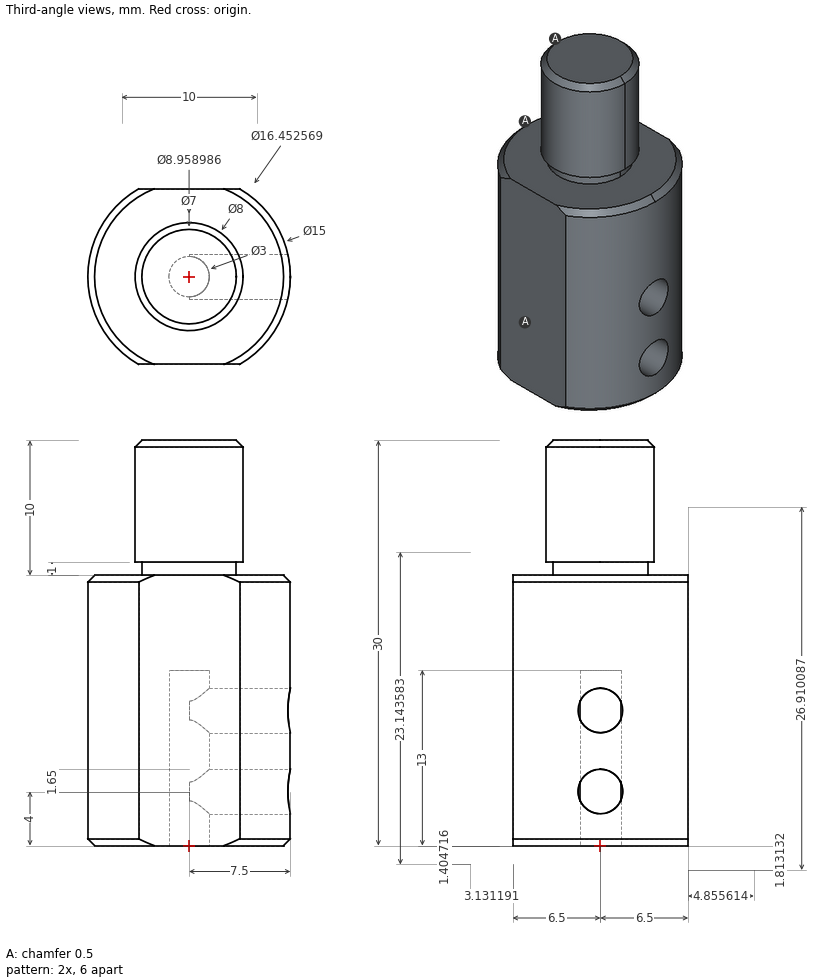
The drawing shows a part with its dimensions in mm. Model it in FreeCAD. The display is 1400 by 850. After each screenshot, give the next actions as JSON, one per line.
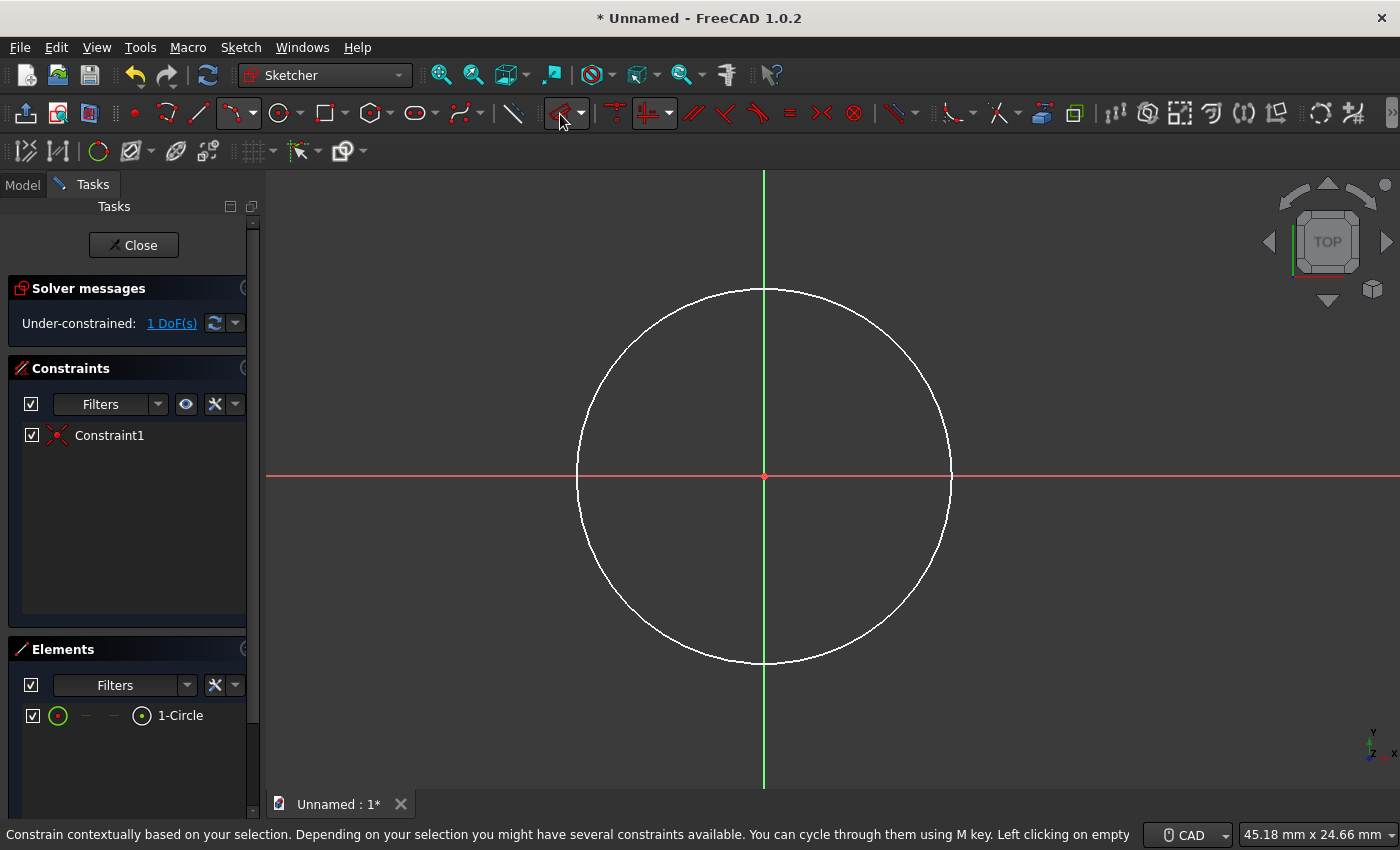
{"action": "left_click", "coordinate": [896, 343]}
{"action": "left_click", "coordinate": [918, 320]}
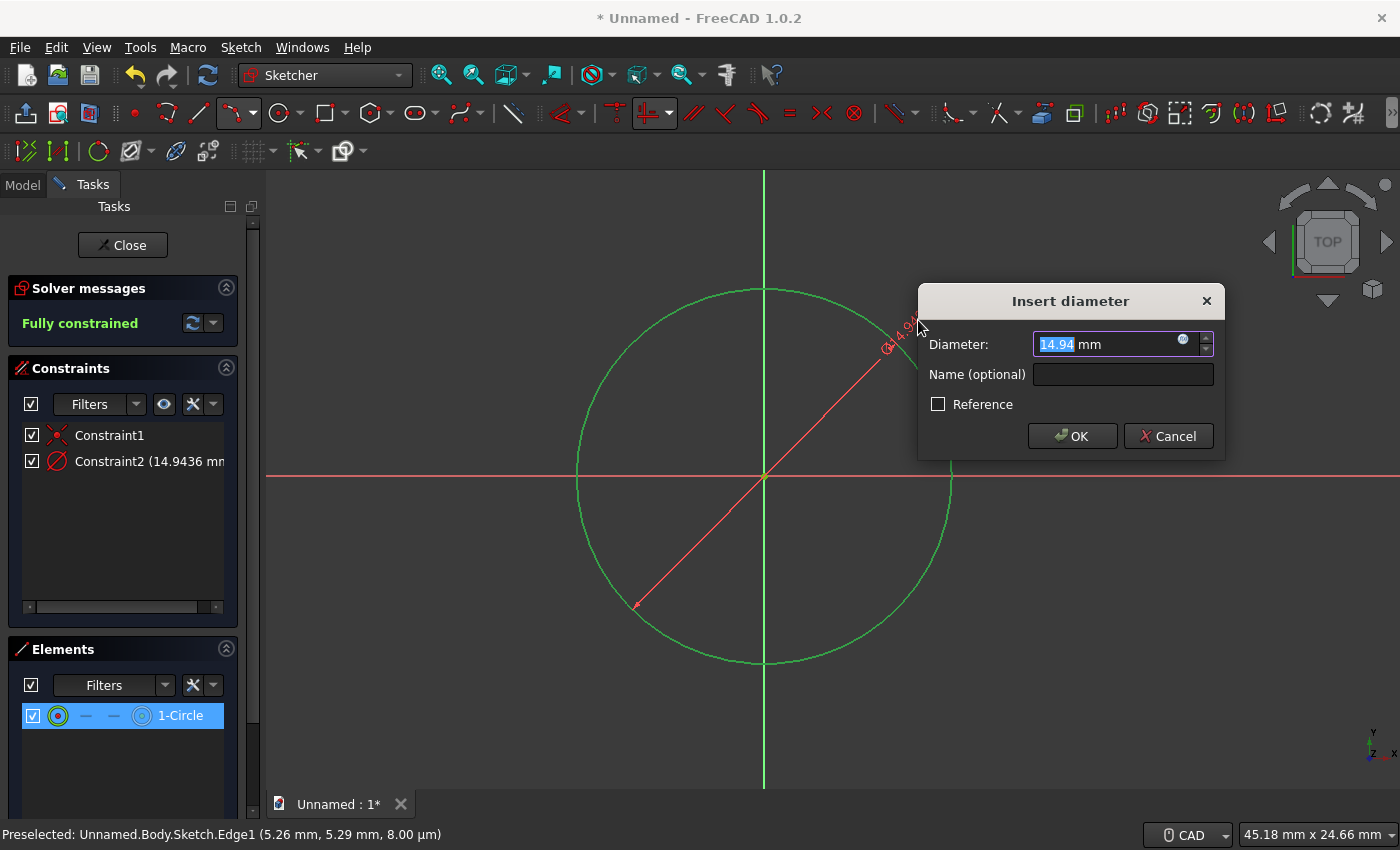
{"action": "type", "text": "15"}
{"action": "key", "text": "Return"}
{"action": "key", "text": "Escape"}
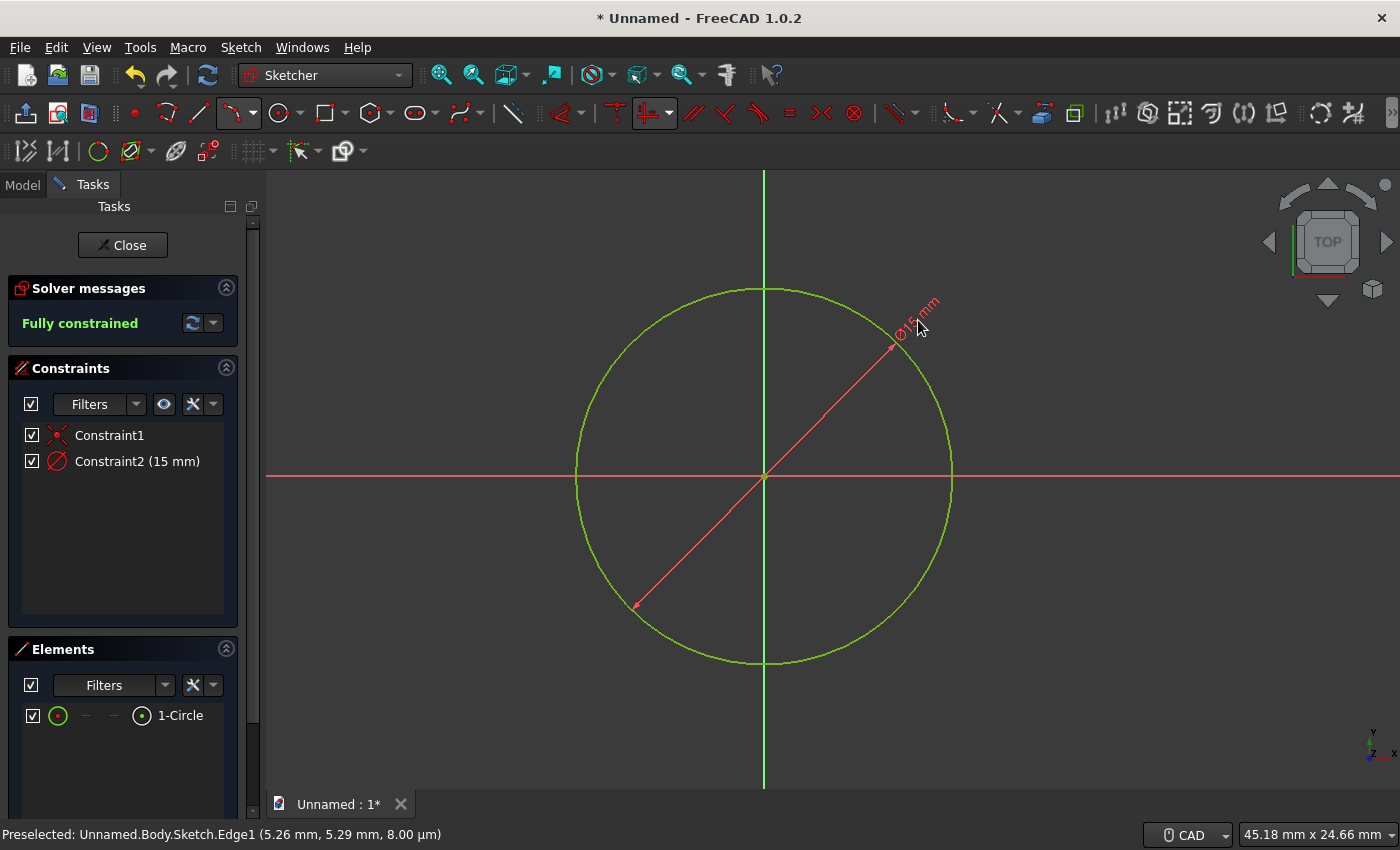
{"action": "left_click", "coordinate": [123, 245]}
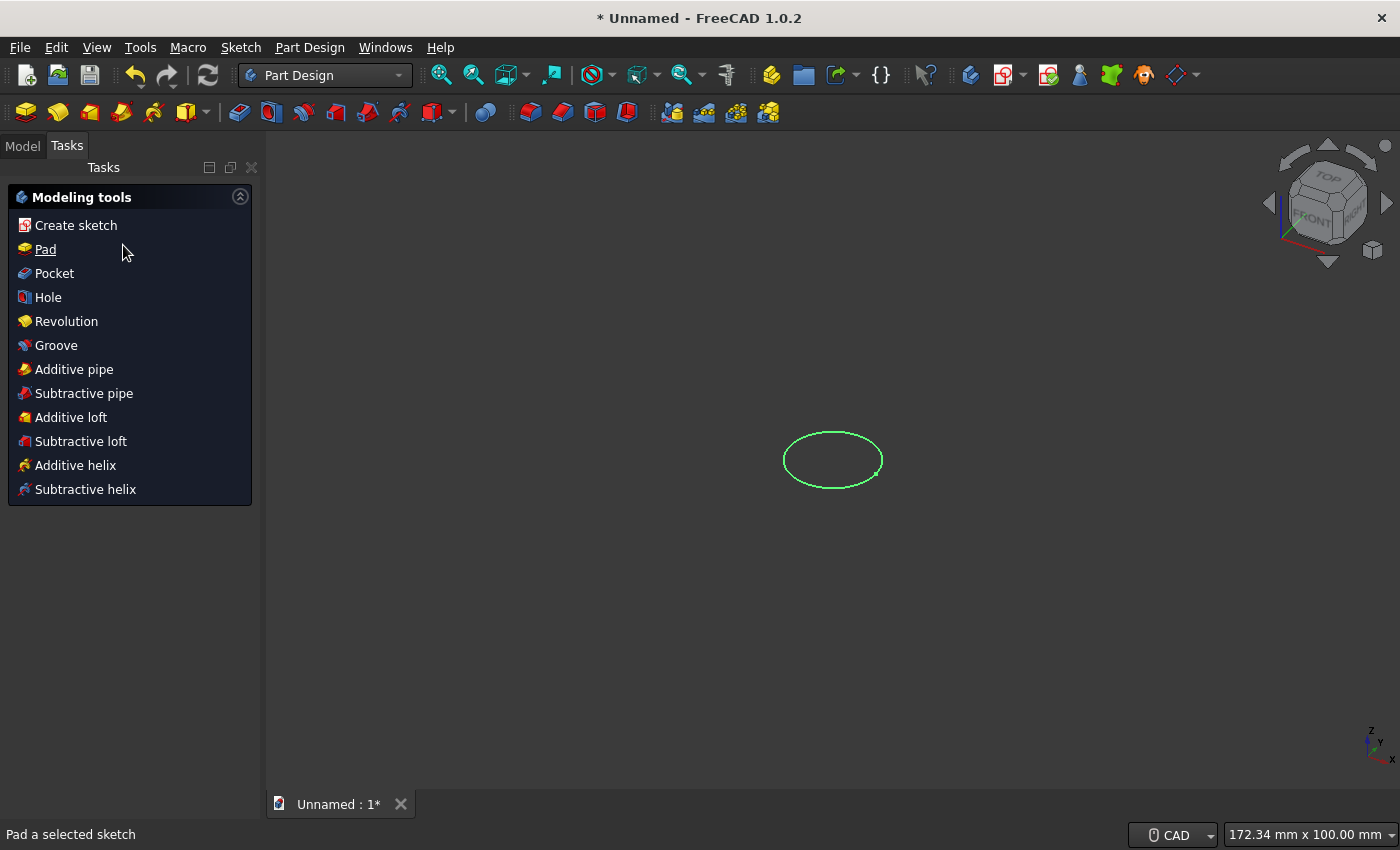
{"action": "left_click", "coordinate": [26, 112]}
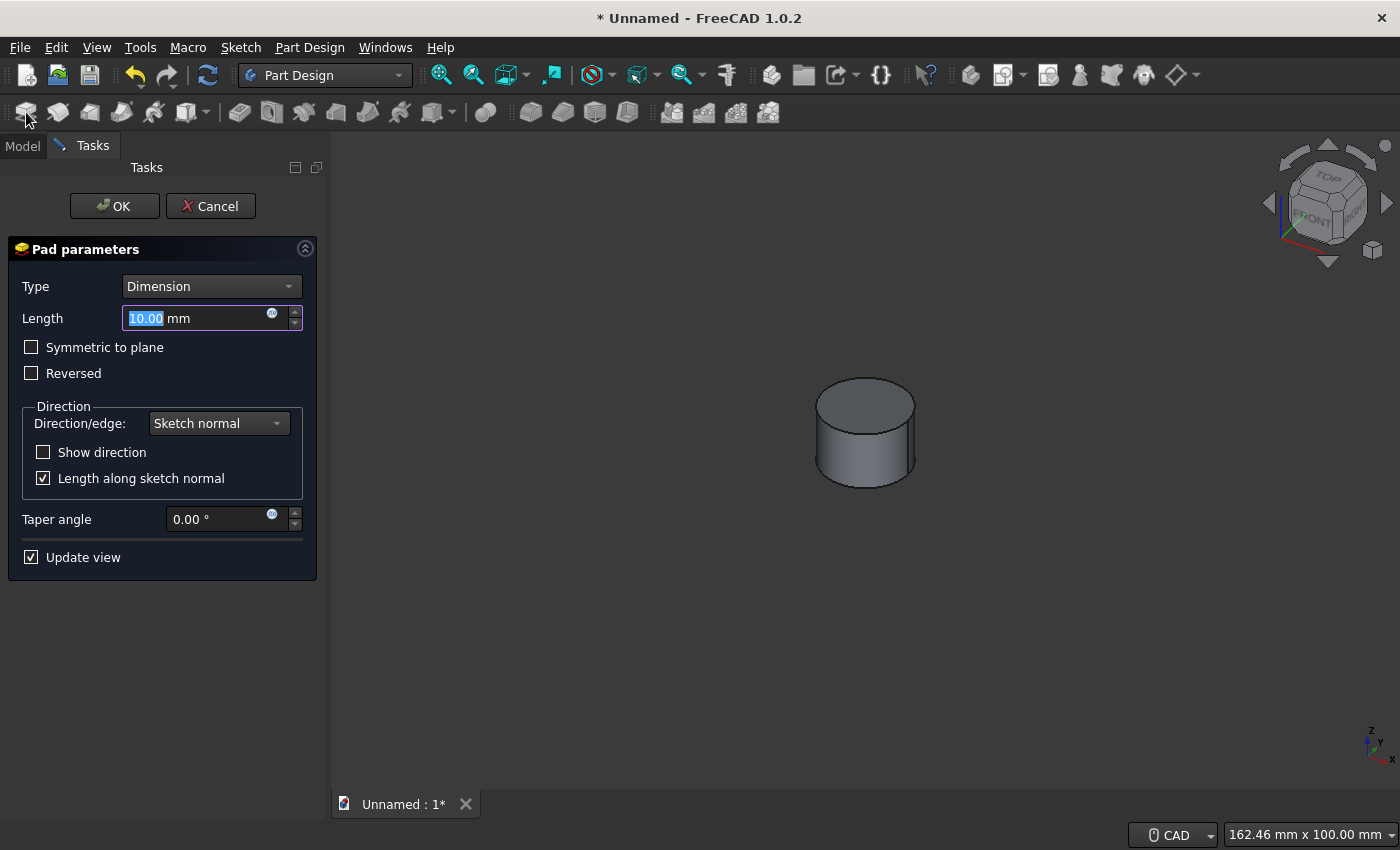
{"action": "type", "text": "30"}
{"action": "key", "text": "Tab"}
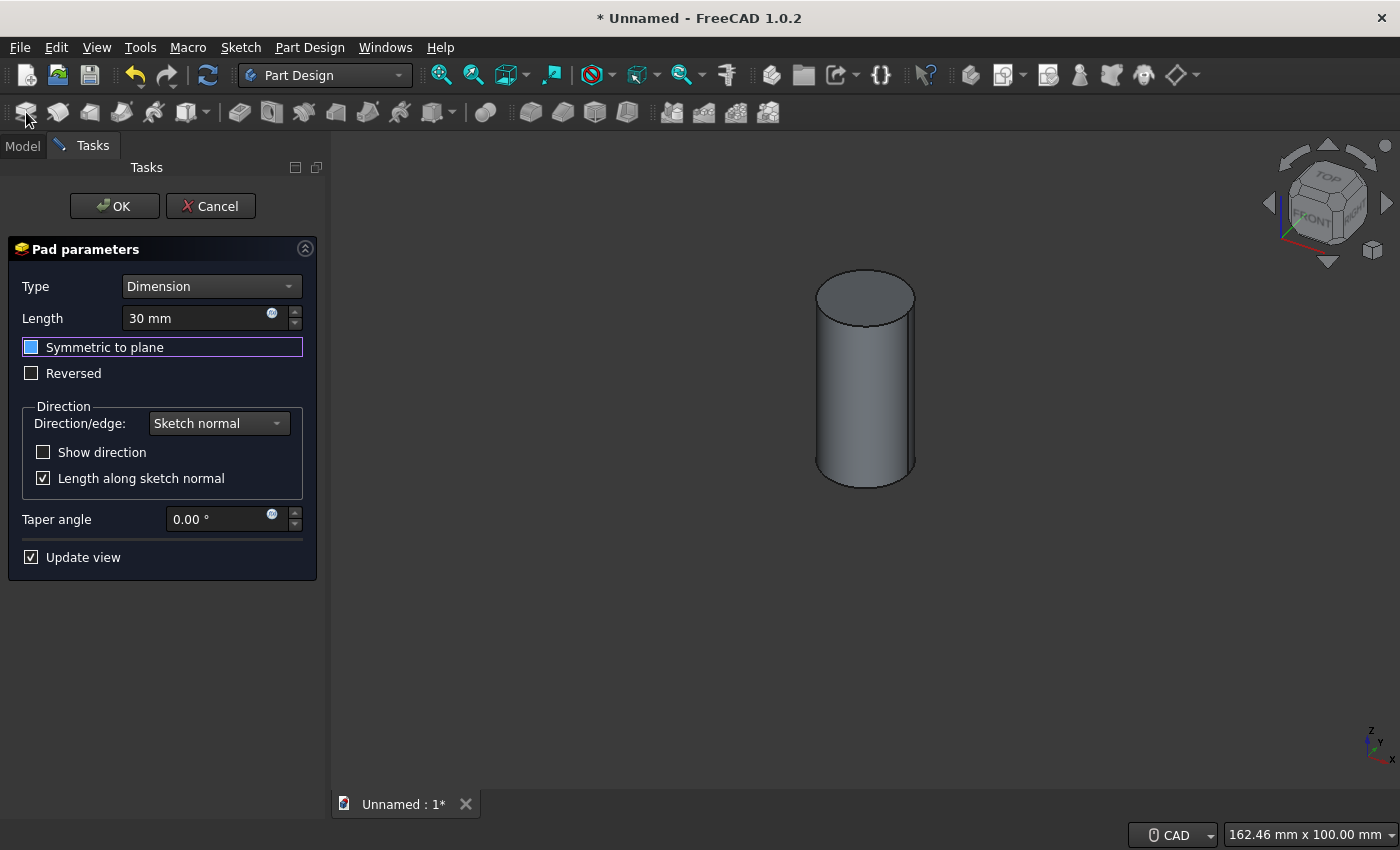
{"action": "left_click", "coordinate": [115, 206]}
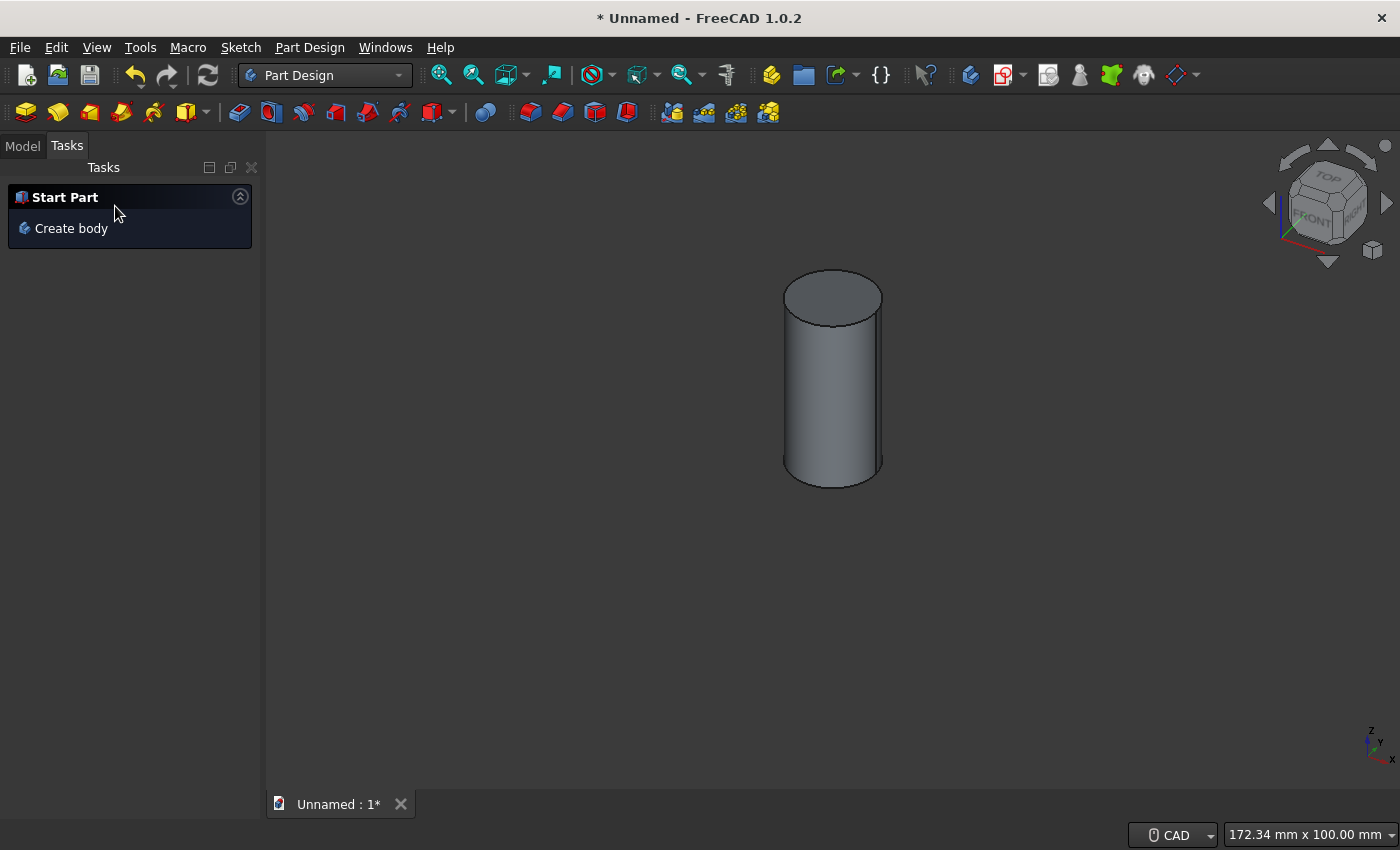
{"action": "left_click", "coordinate": [442, 76]}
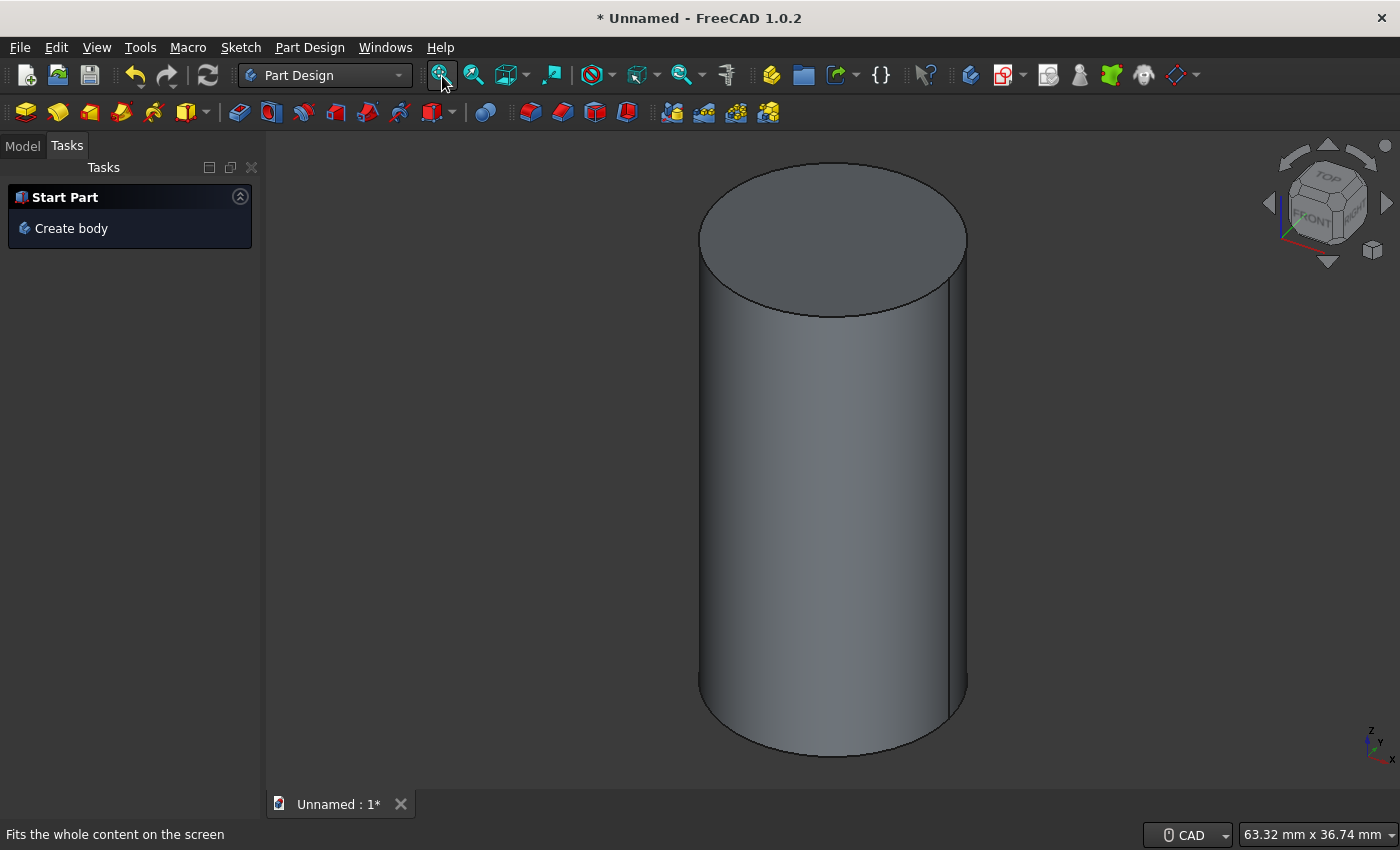
{"action": "left_click", "coordinate": [833, 239]}